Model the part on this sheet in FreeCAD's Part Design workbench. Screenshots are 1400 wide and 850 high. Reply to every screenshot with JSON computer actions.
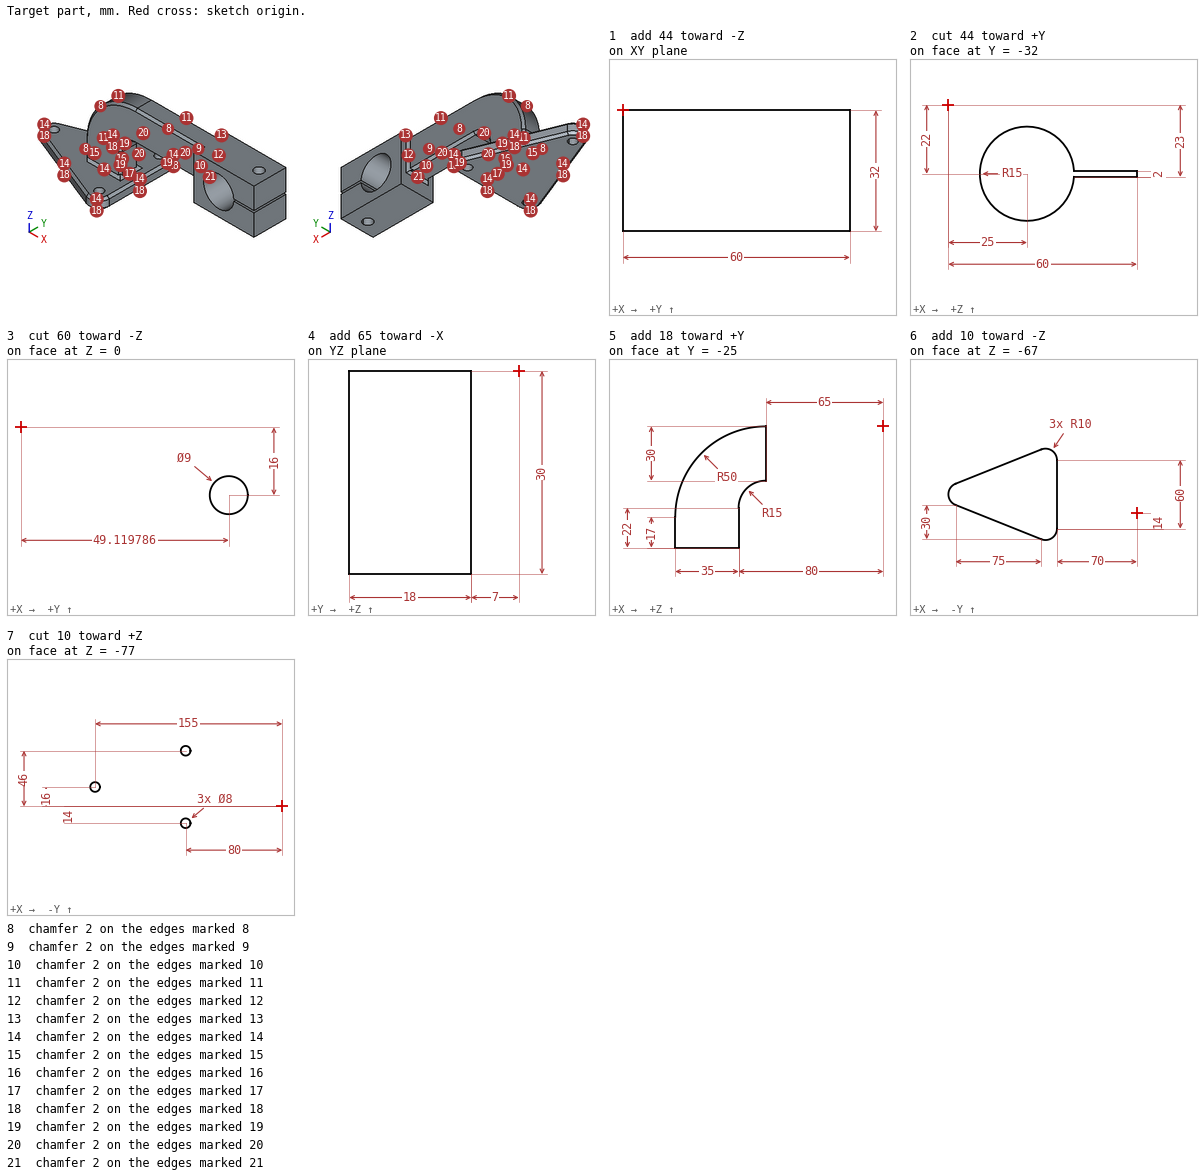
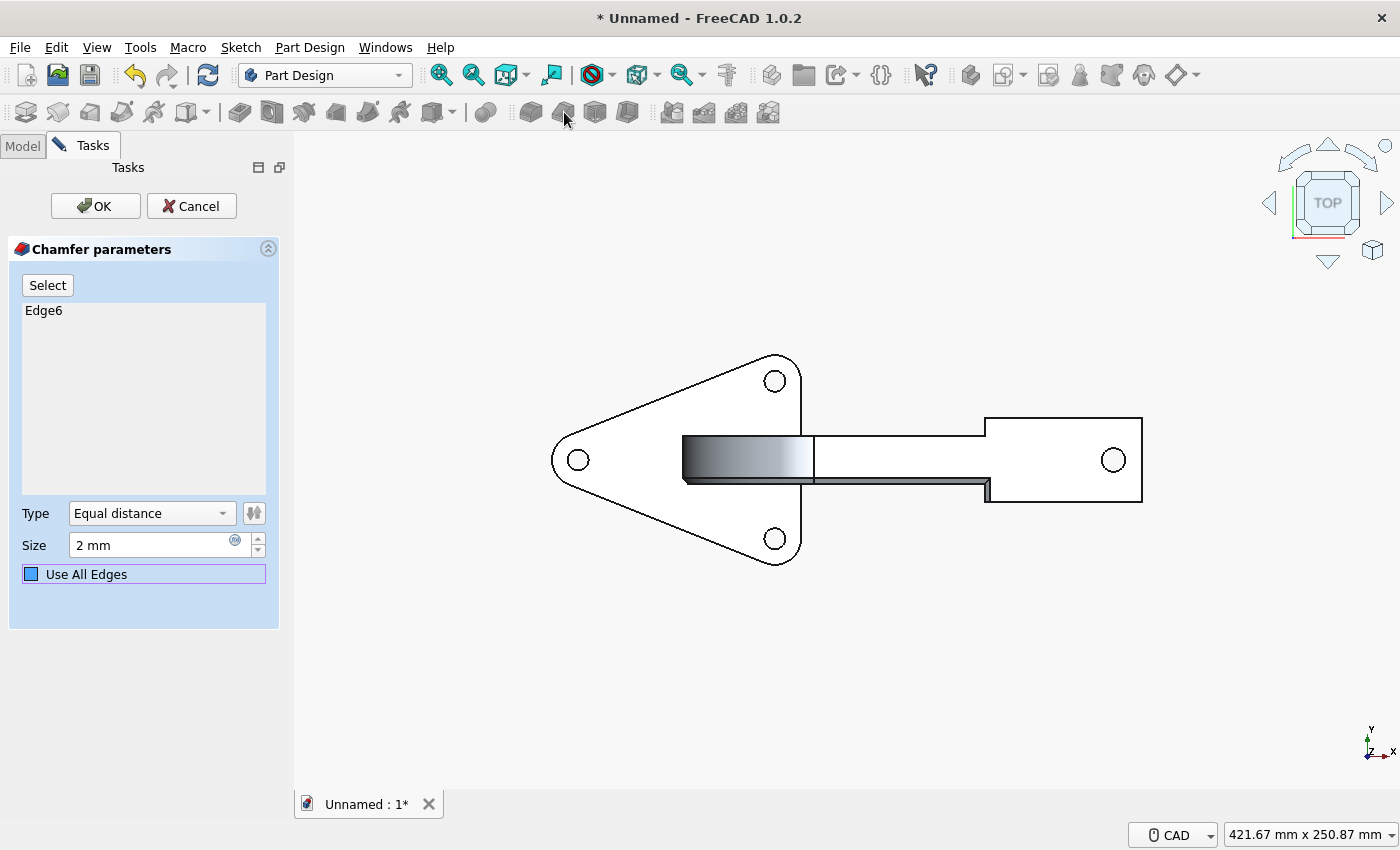
{"action": "left_click", "coordinate": [96, 206]}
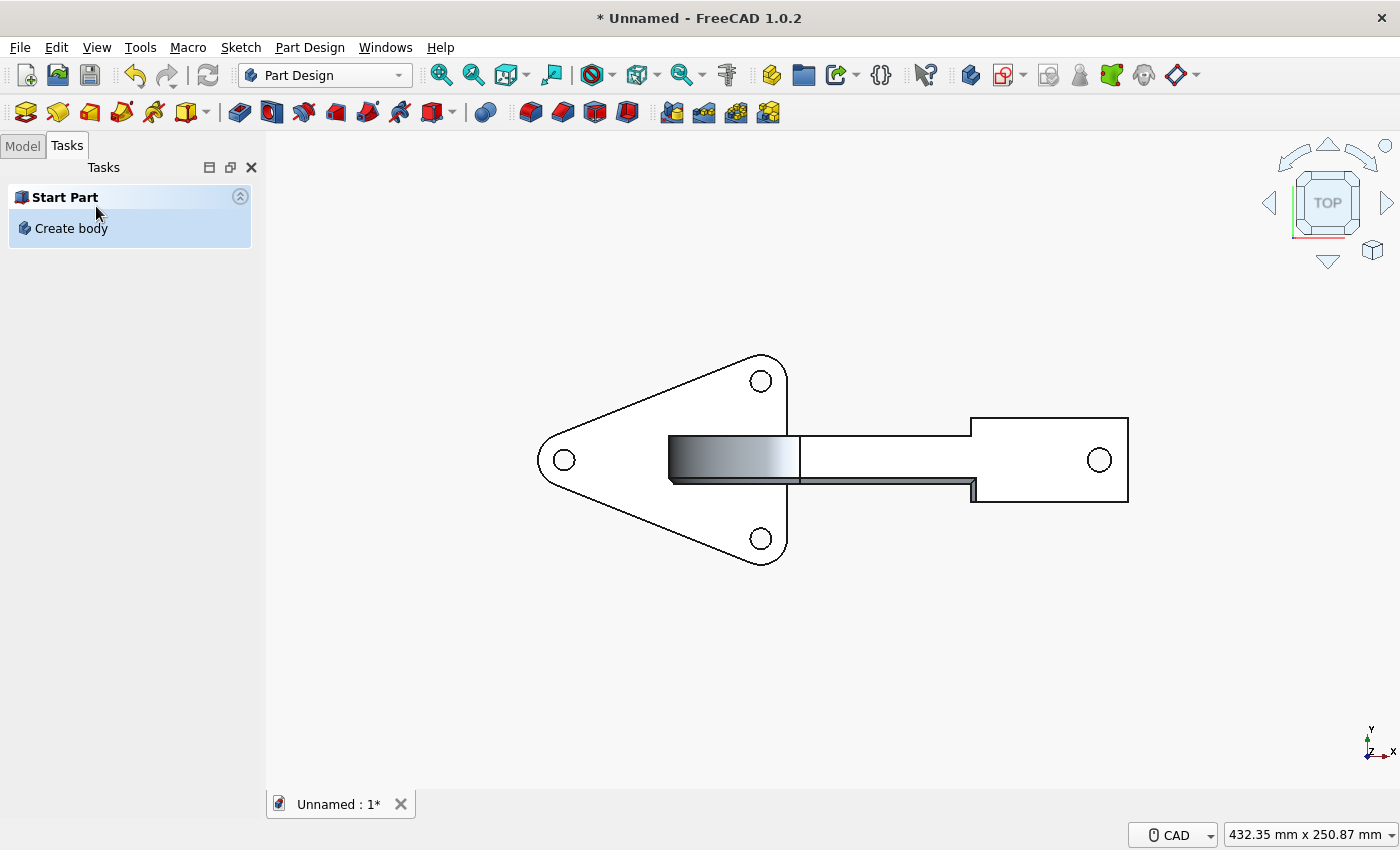
{"action": "key", "text": "0"}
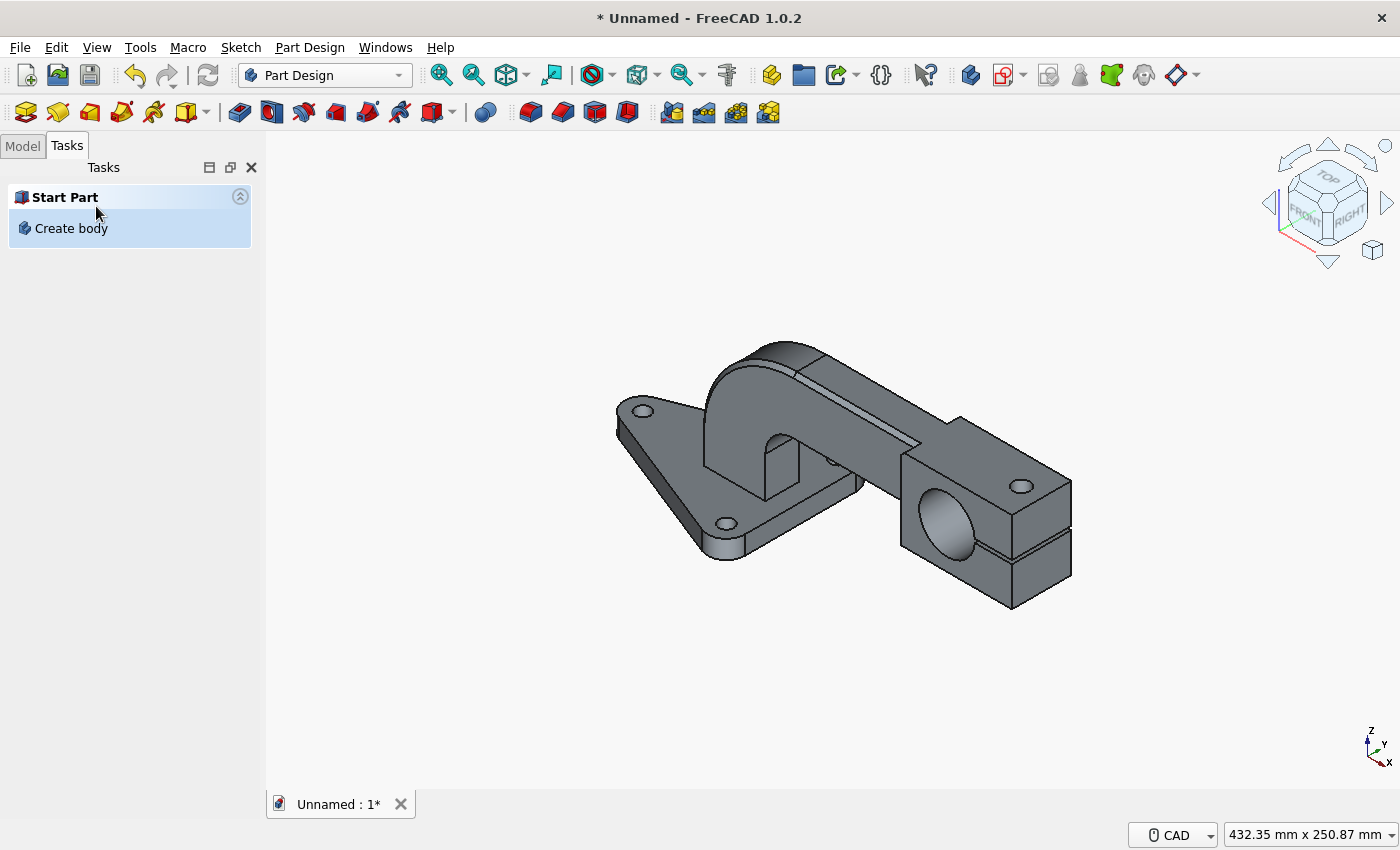
{"action": "key", "text": "2"}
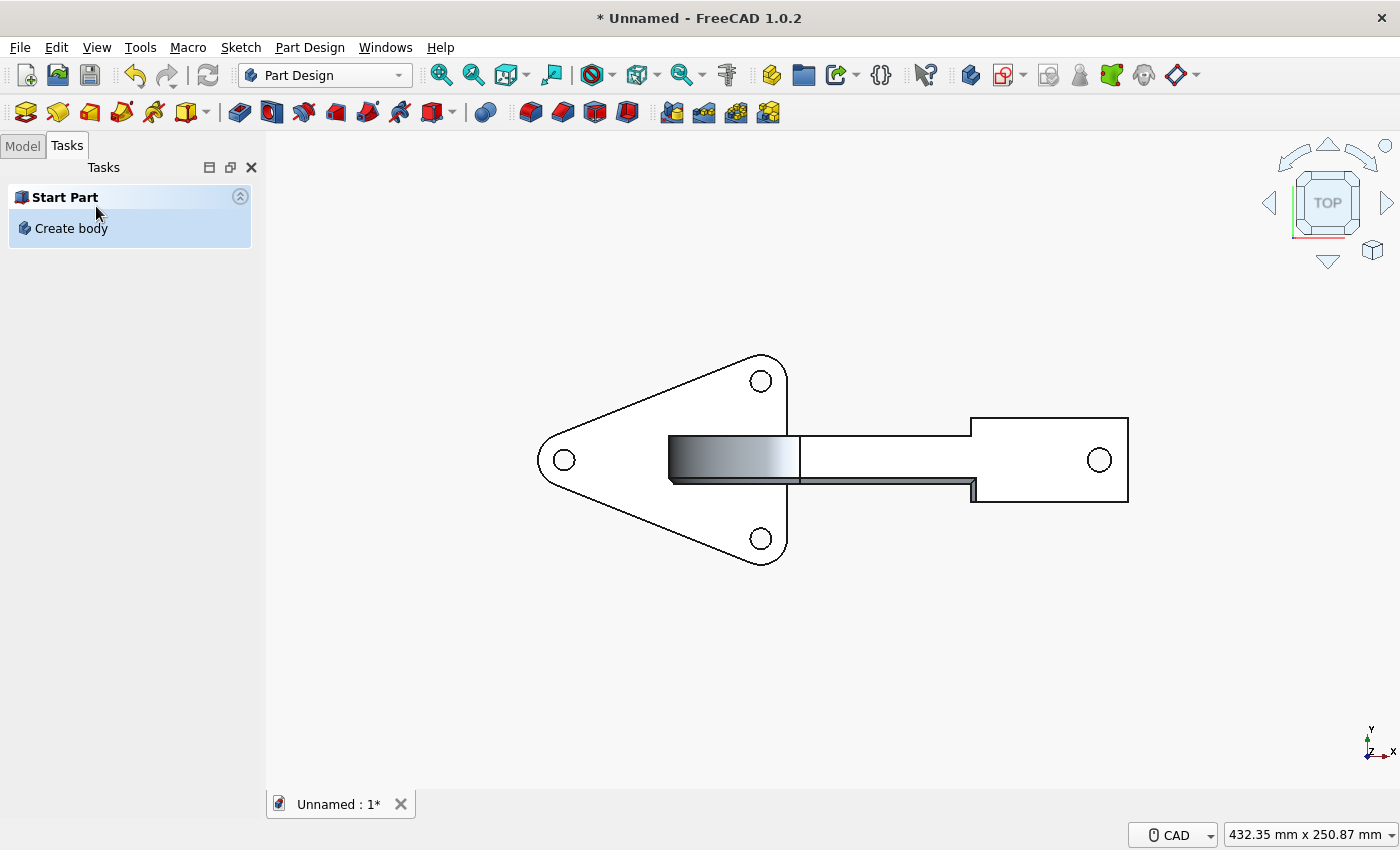
{"action": "key", "text": "1"}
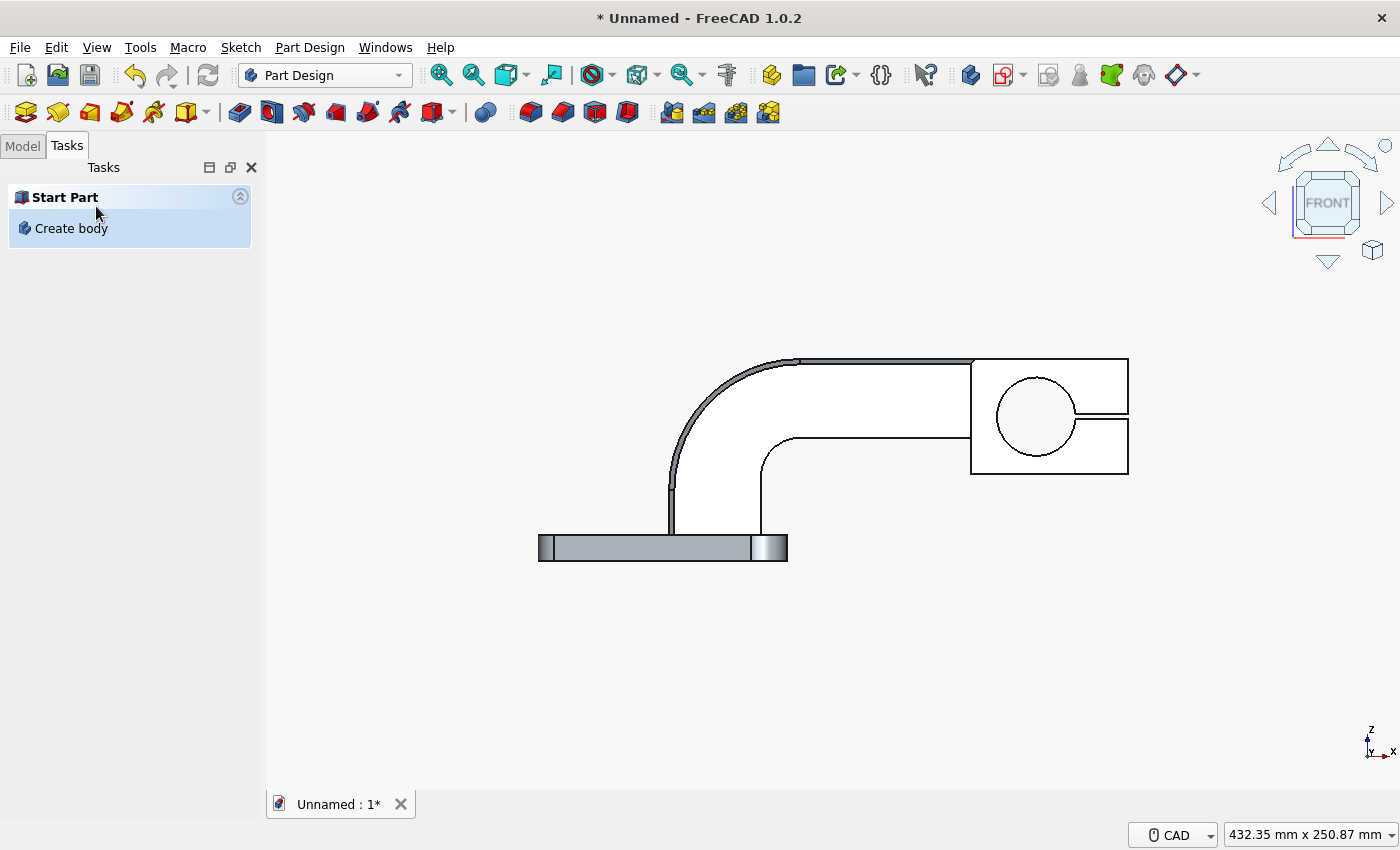
{"action": "key", "text": "3"}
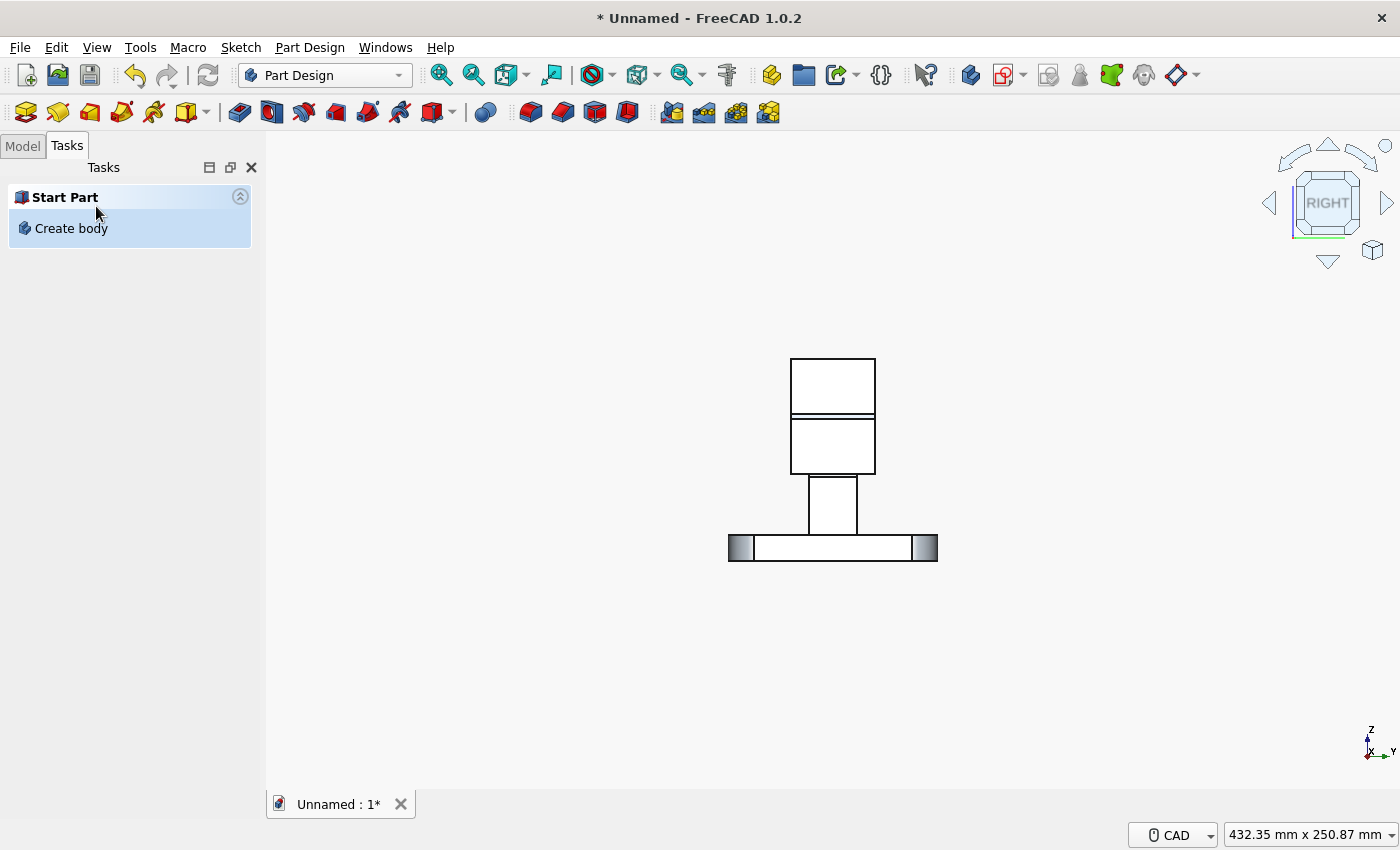
{"action": "left_click", "coordinate": [442, 76]}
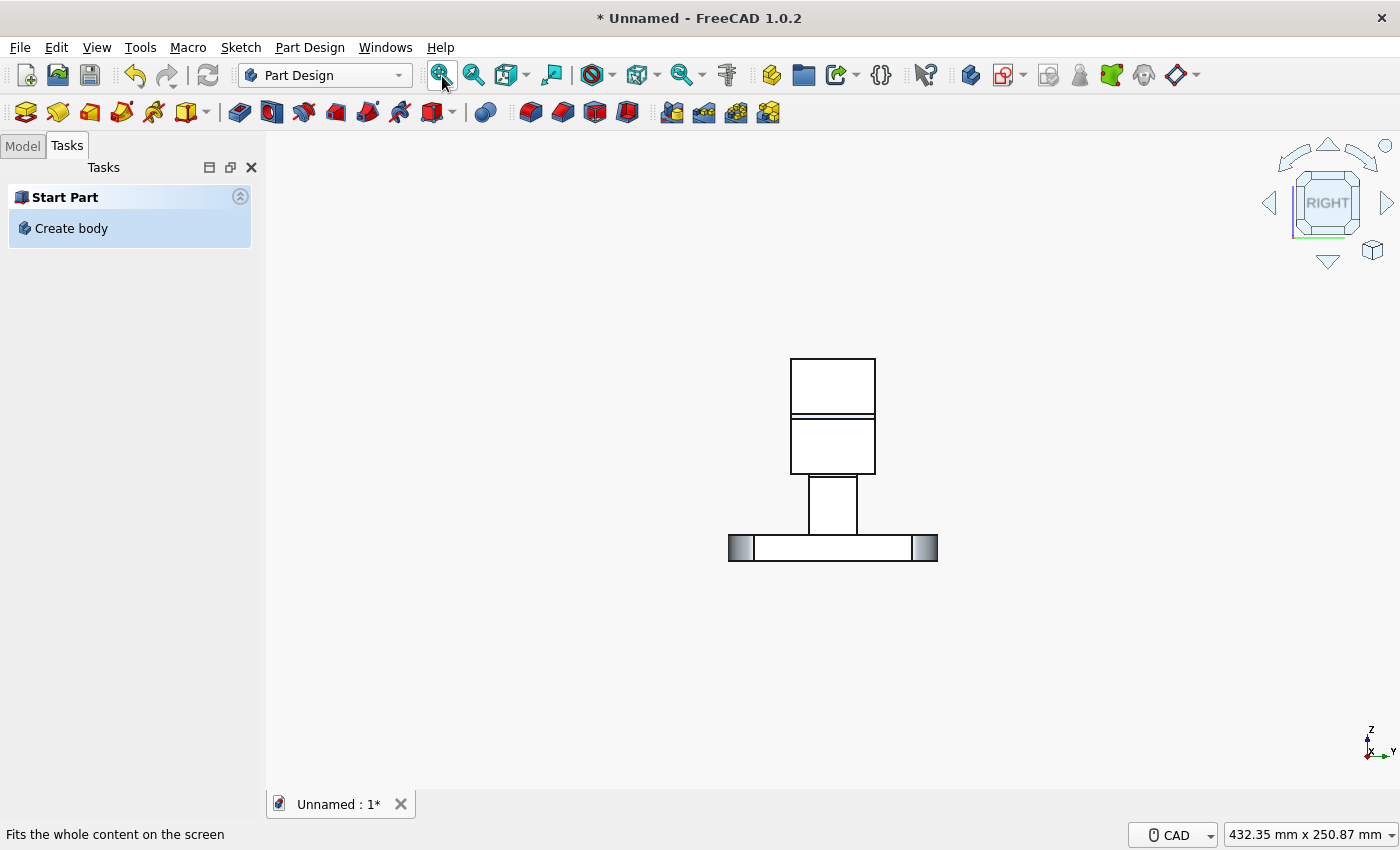
{"action": "key", "text": "5"}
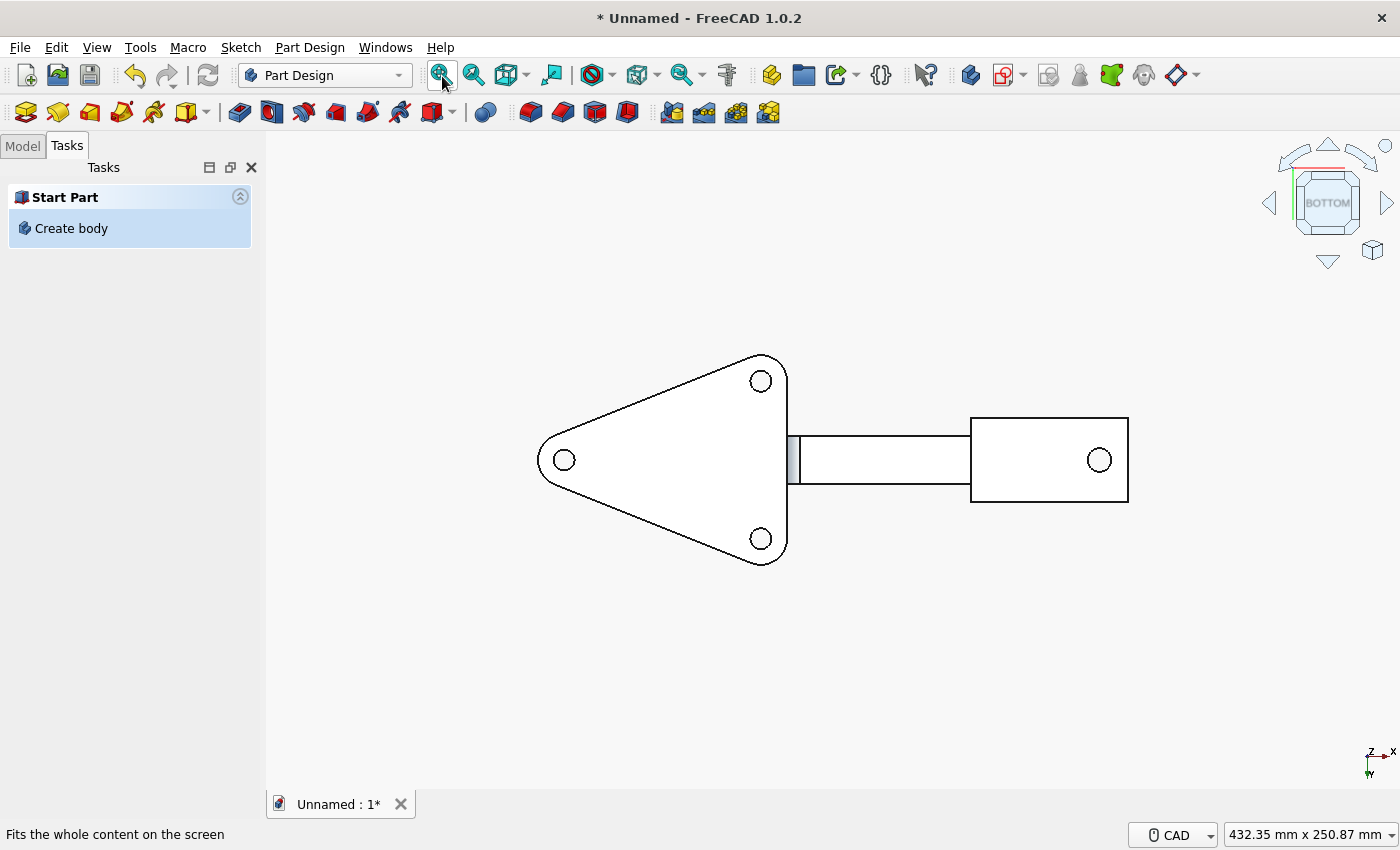
{"action": "key", "text": "4"}